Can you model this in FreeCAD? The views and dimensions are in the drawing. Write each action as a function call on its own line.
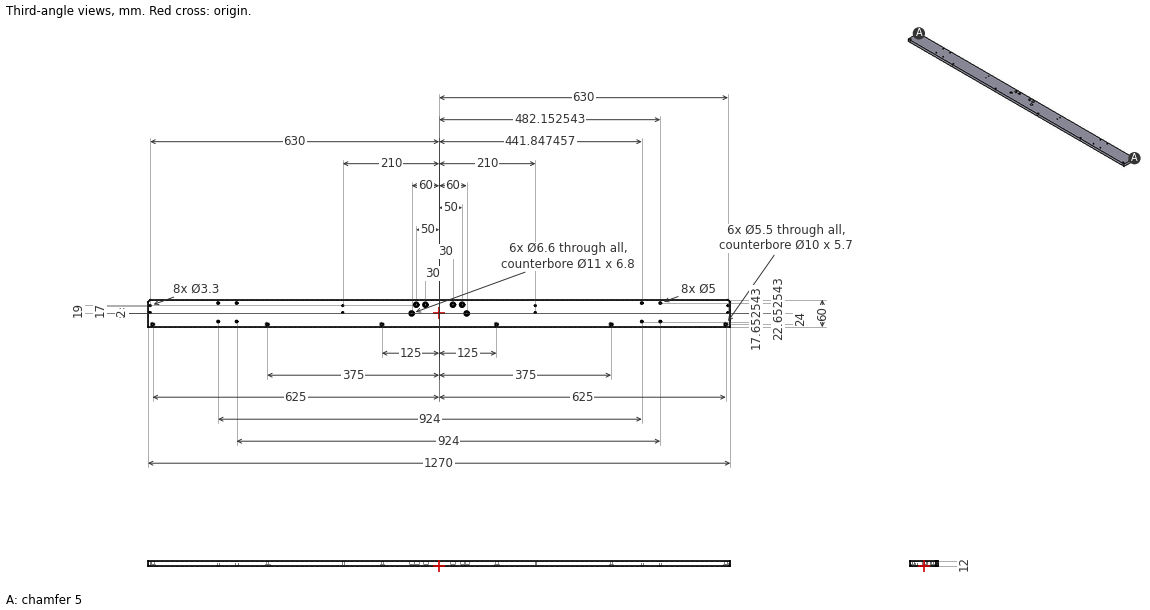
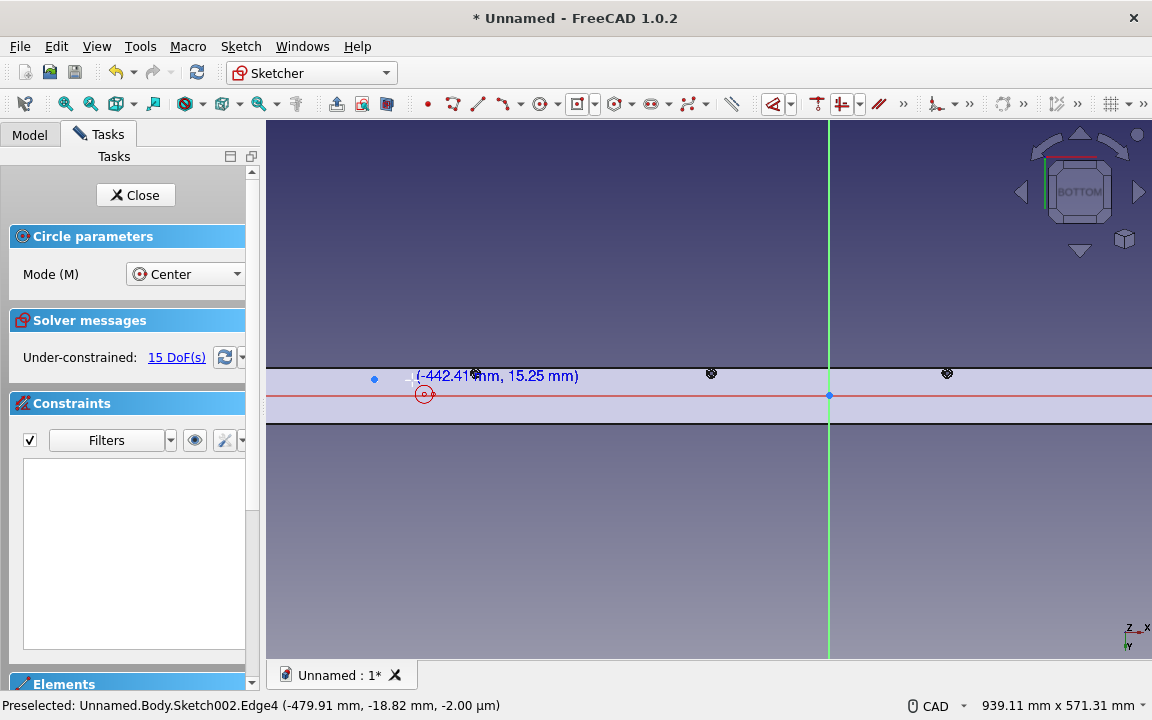
click(412, 379)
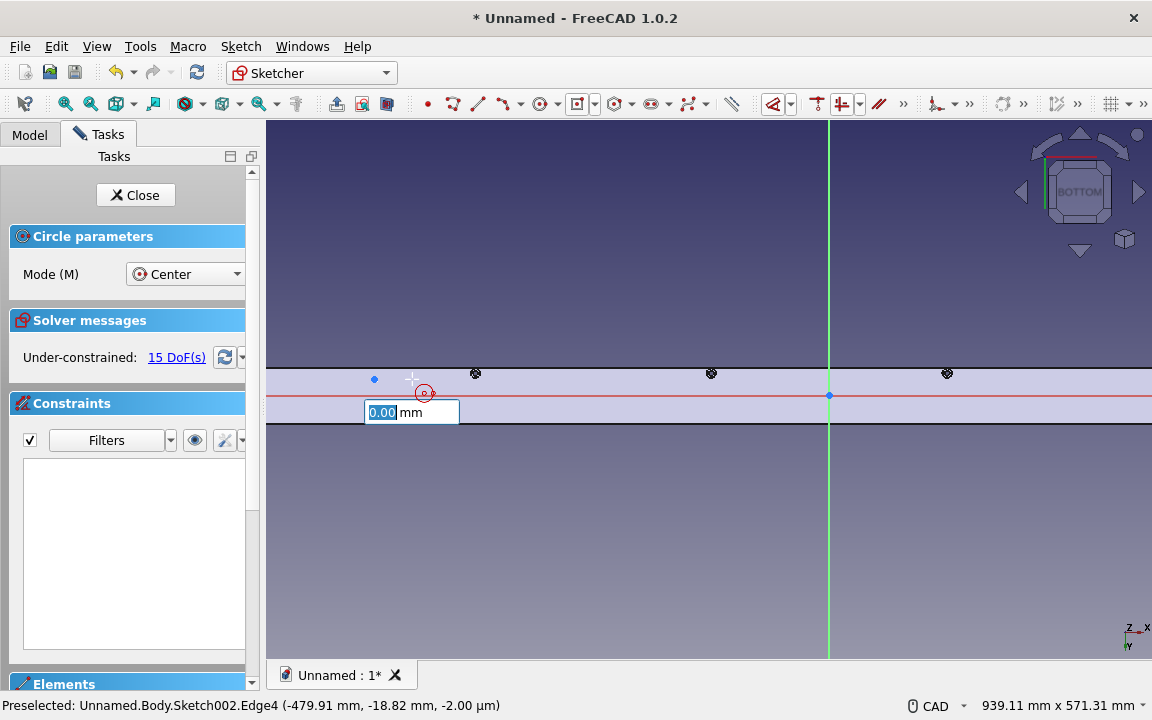
scroll(414, 377, up, 10)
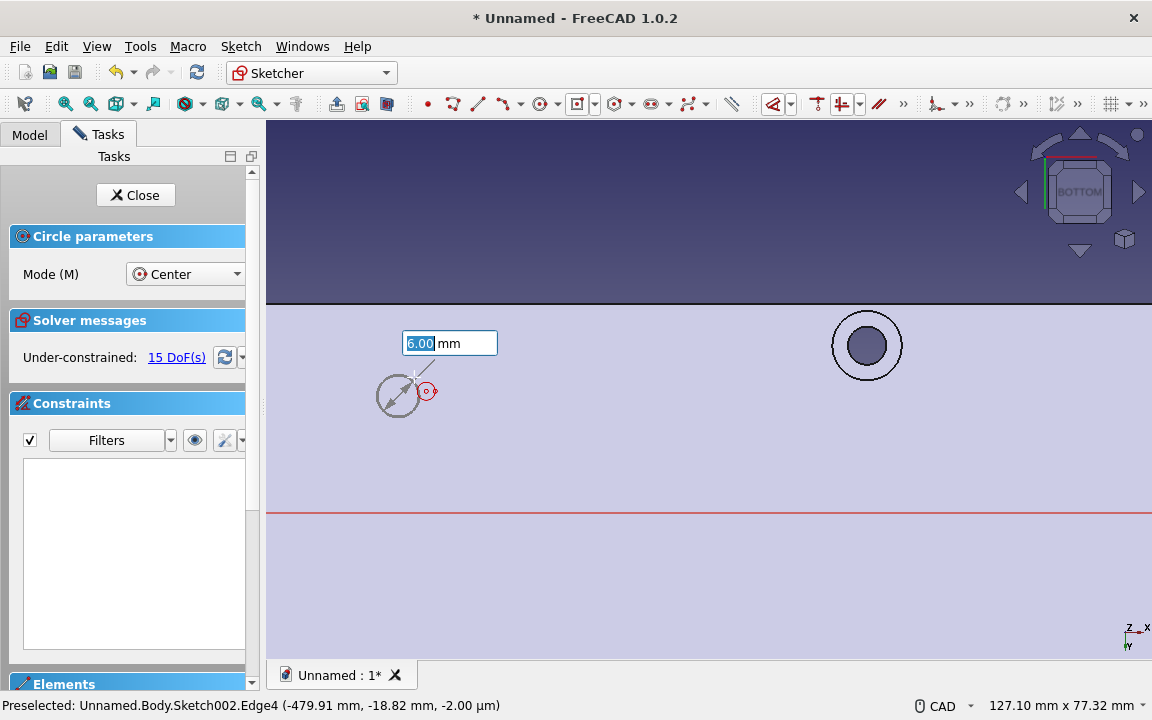
click(413, 378)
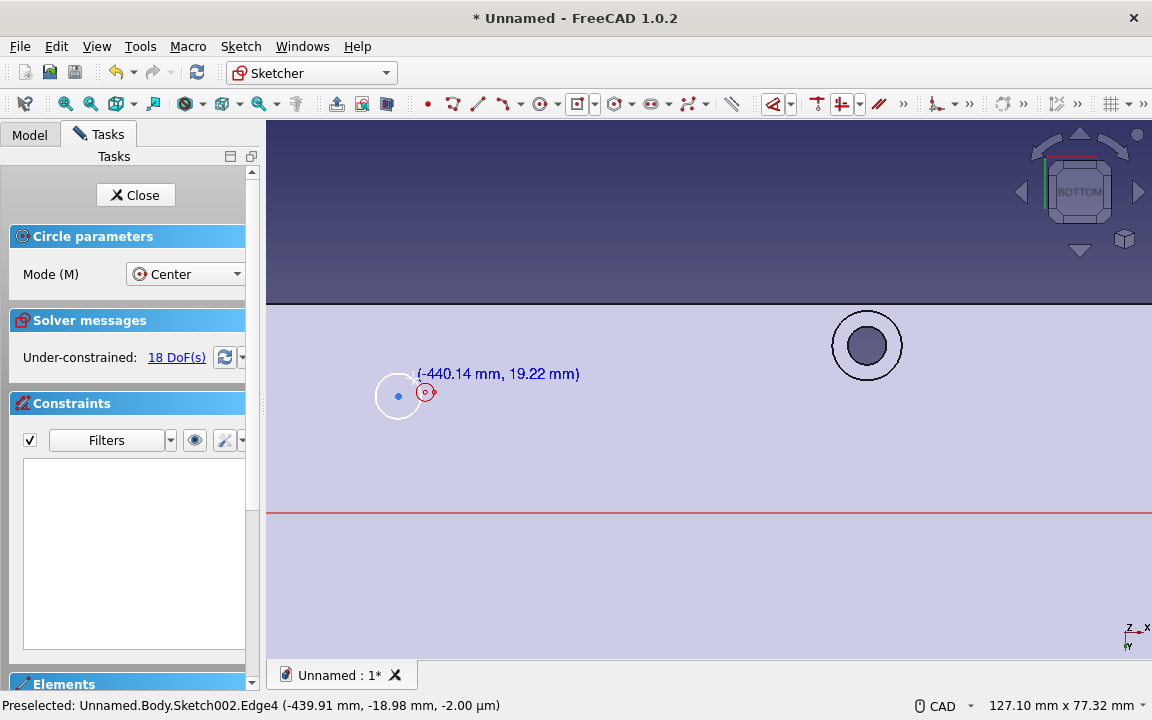
scroll(413, 378, down, 13)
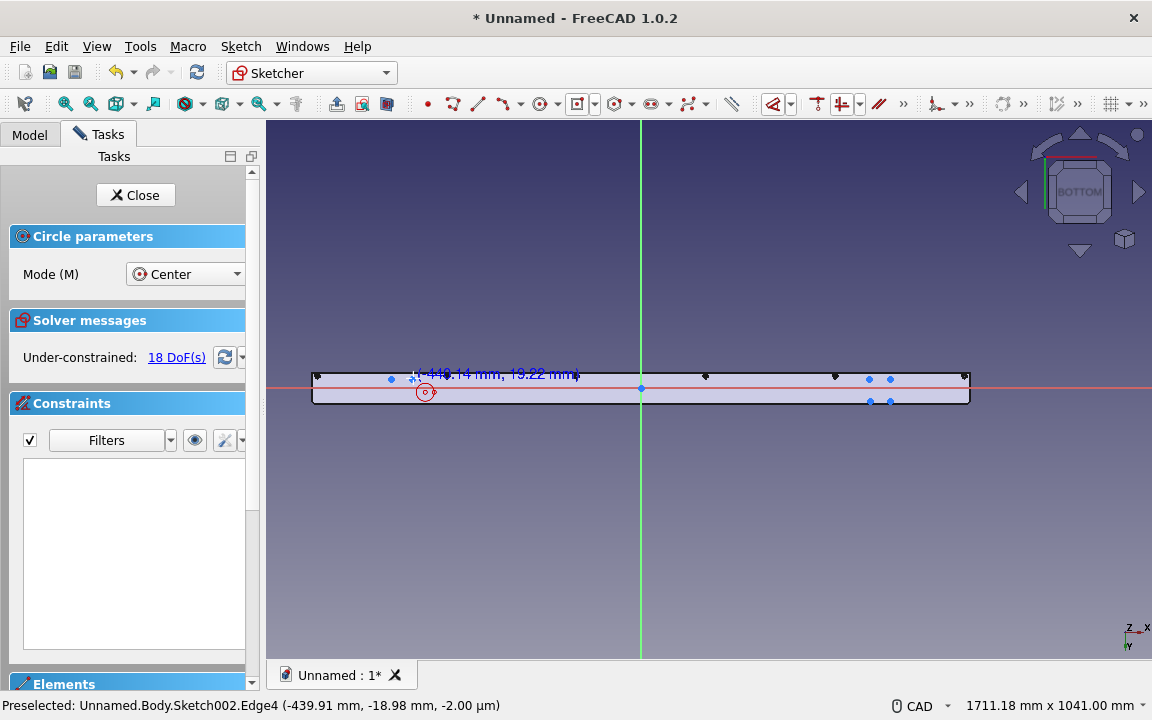
scroll(412, 400, up, 15)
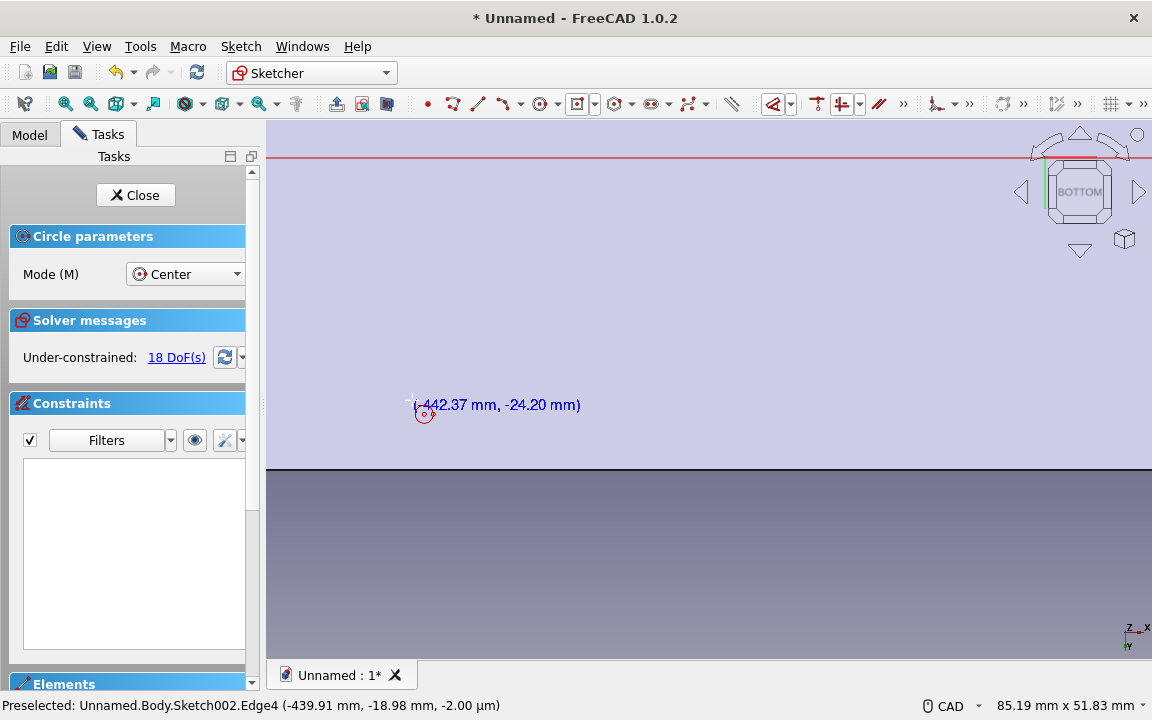
scroll(412, 400, down, 15)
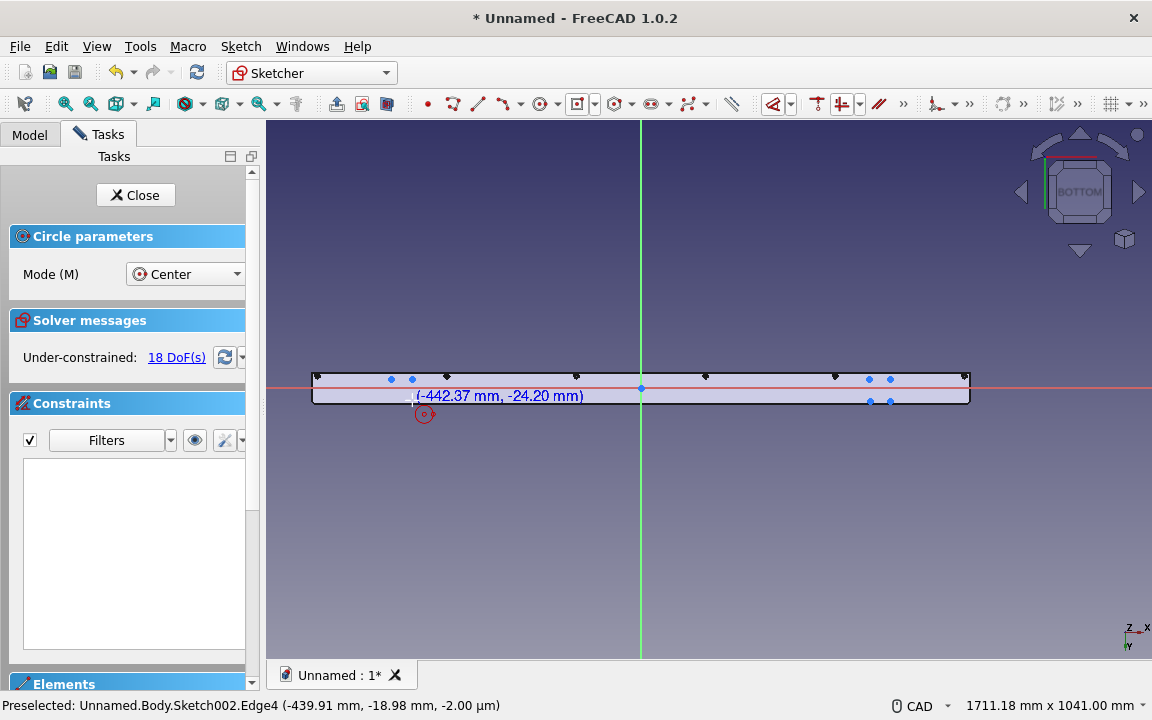
scroll(412, 400, up, 2)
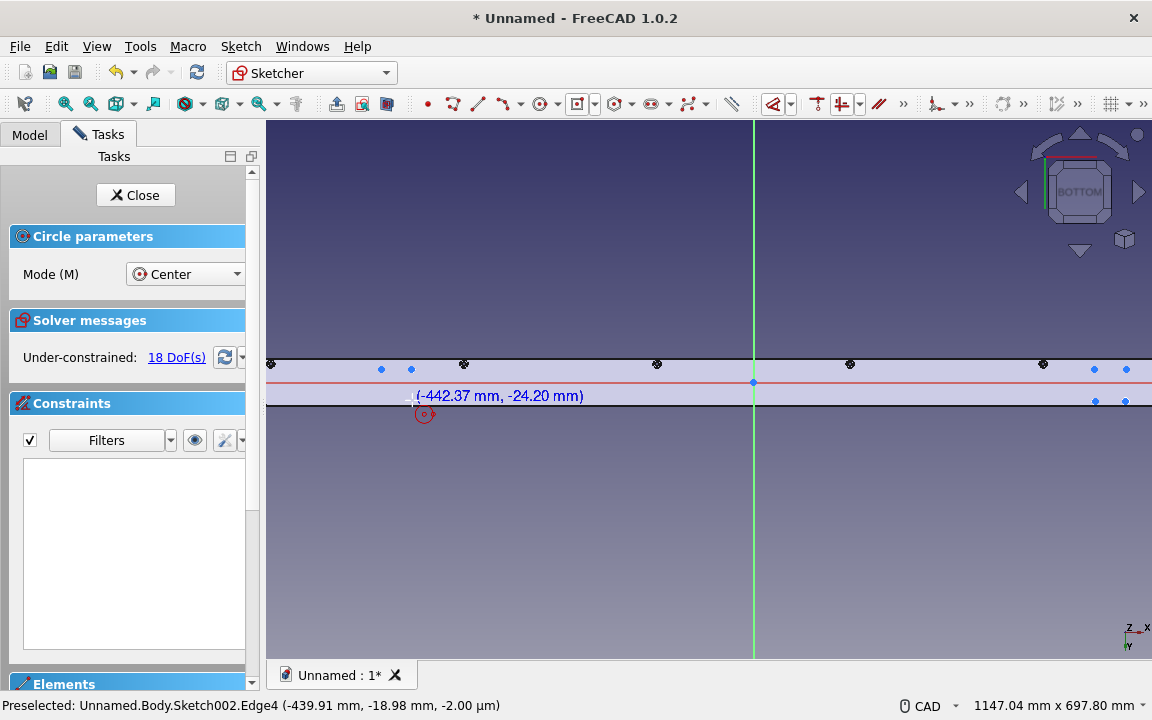
click(412, 400)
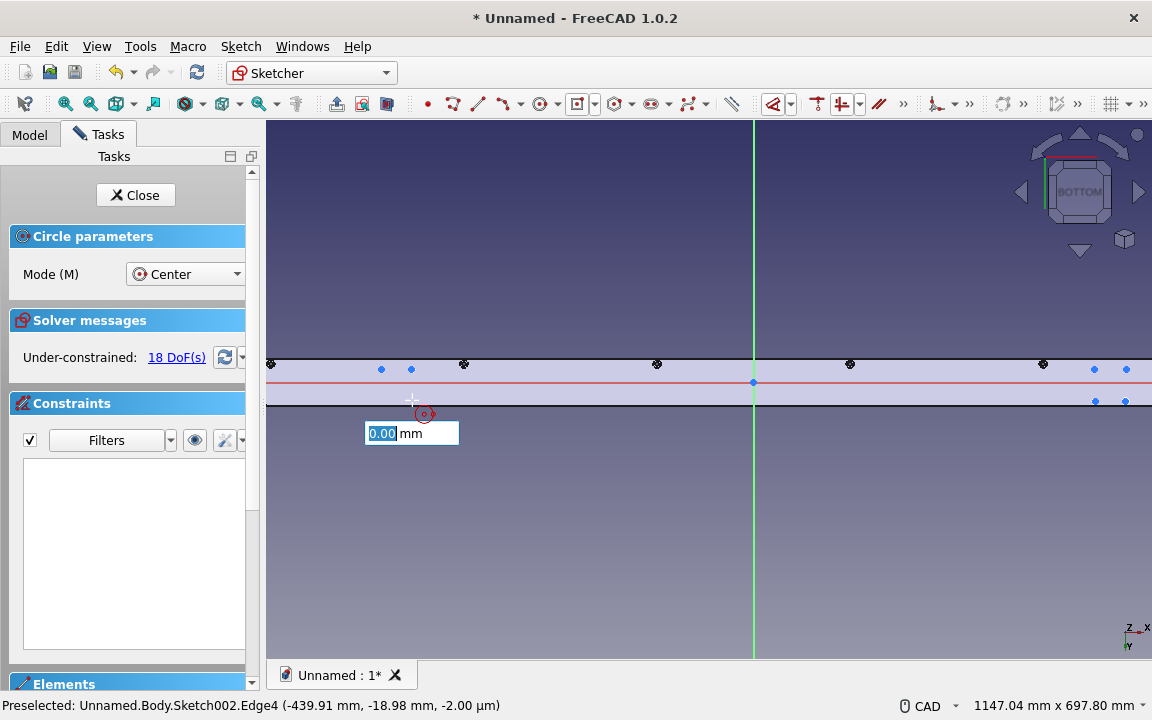
scroll(414, 399, up, 11)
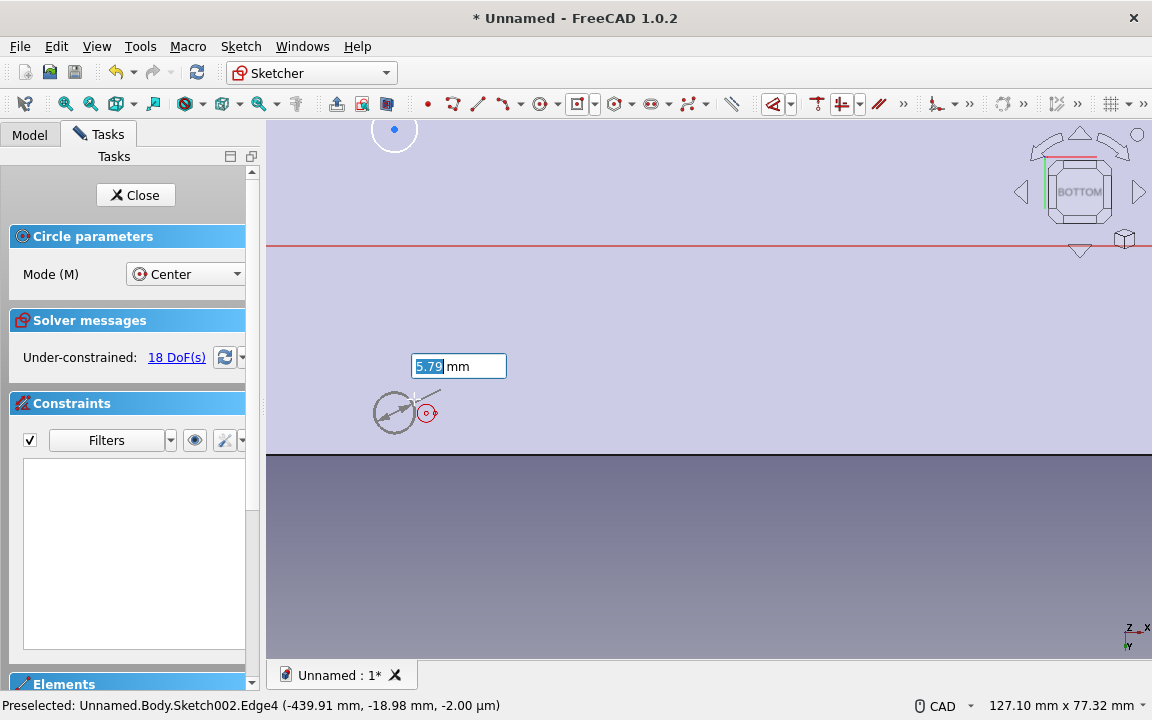
click(410, 392)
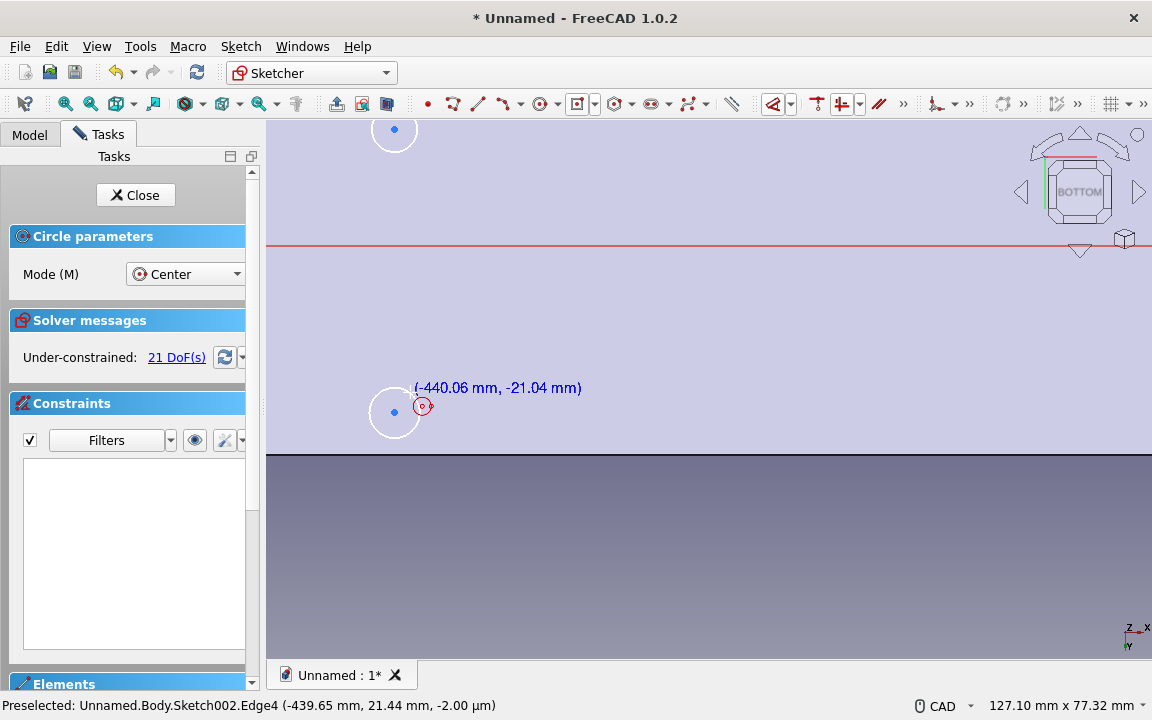
scroll(413, 400, down, 13)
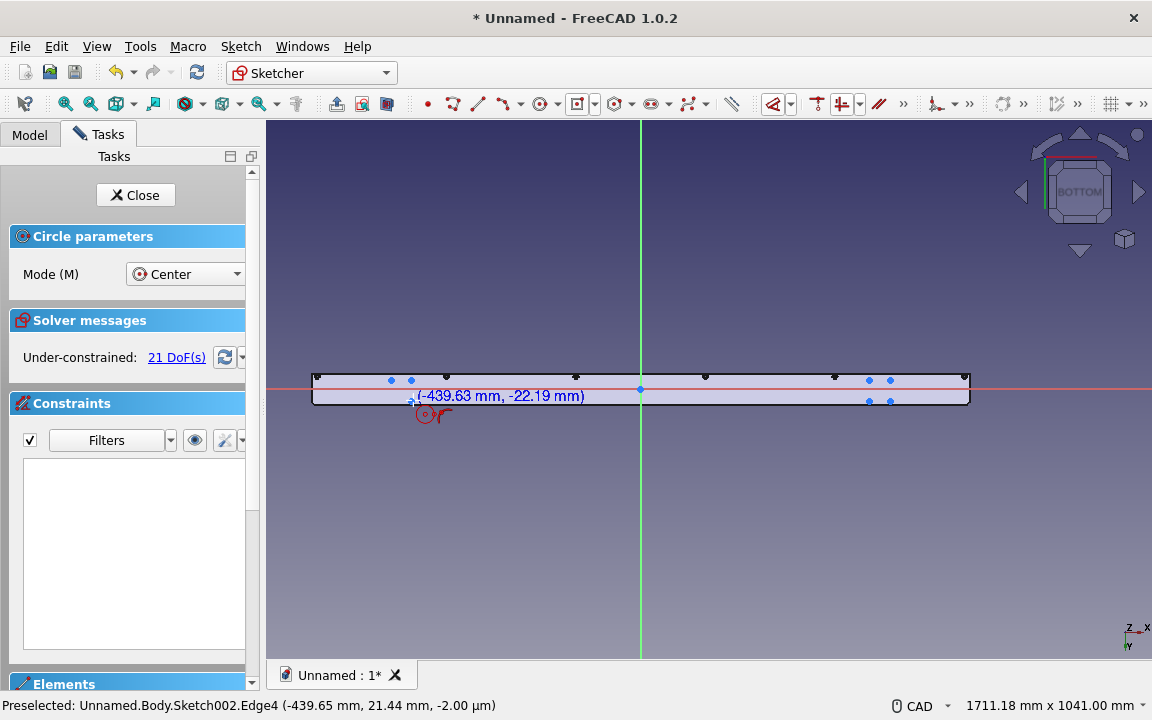
scroll(391, 401, up, 15)